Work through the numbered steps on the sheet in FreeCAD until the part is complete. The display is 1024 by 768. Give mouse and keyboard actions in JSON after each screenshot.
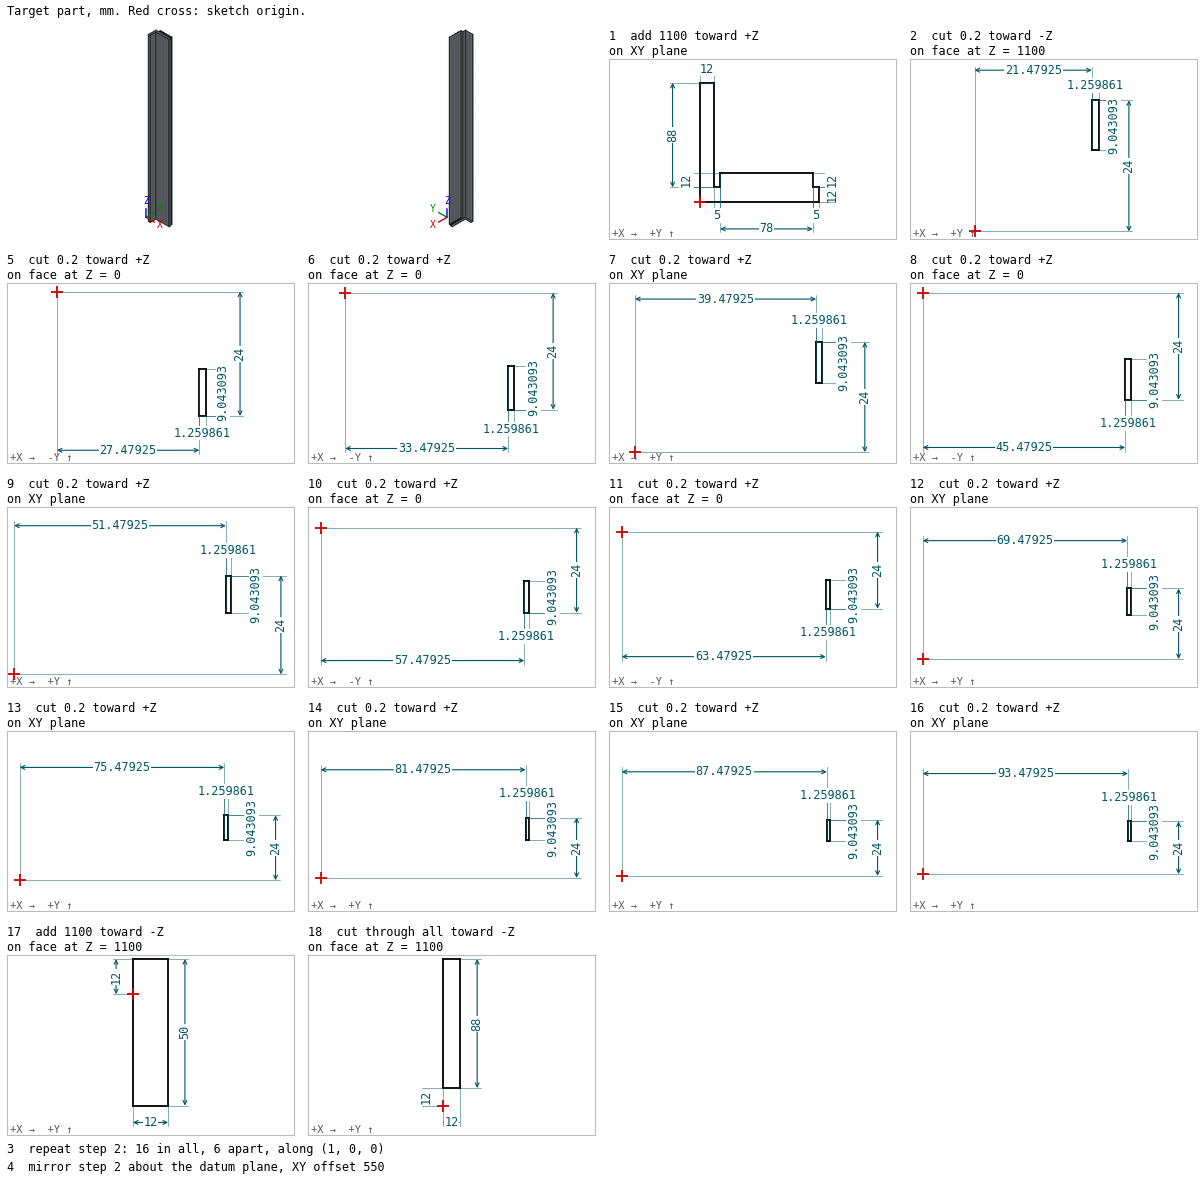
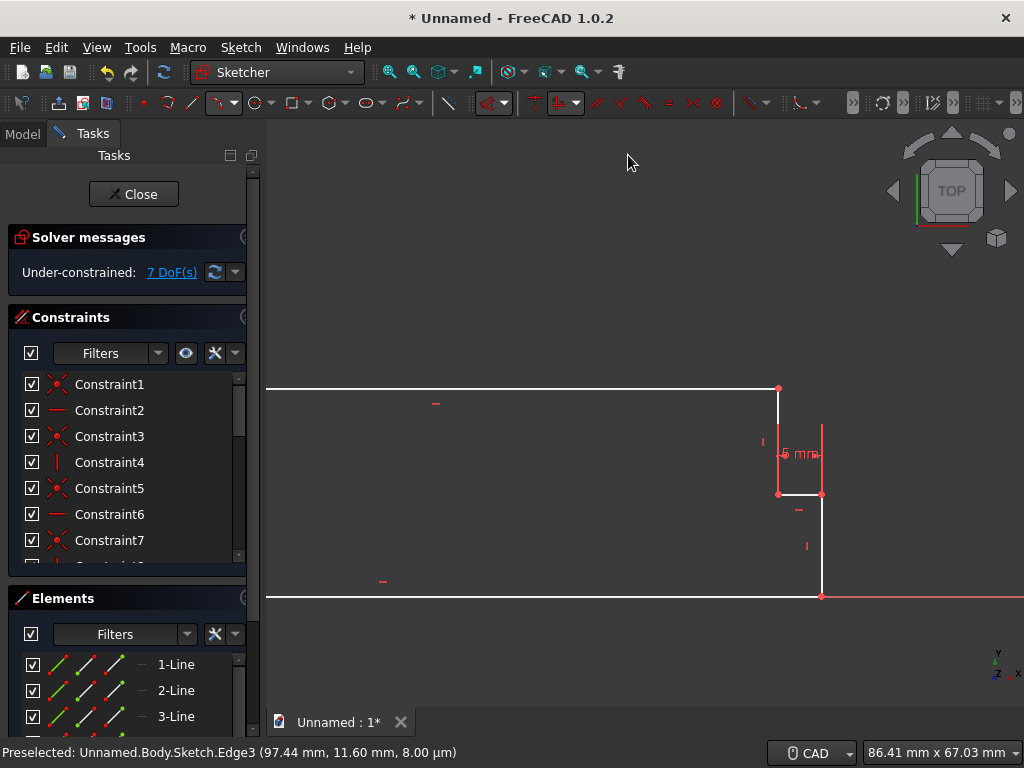
{"action": "scroll", "coordinate": [734, 621], "scroll_direction": "down", "scroll_amount": 4}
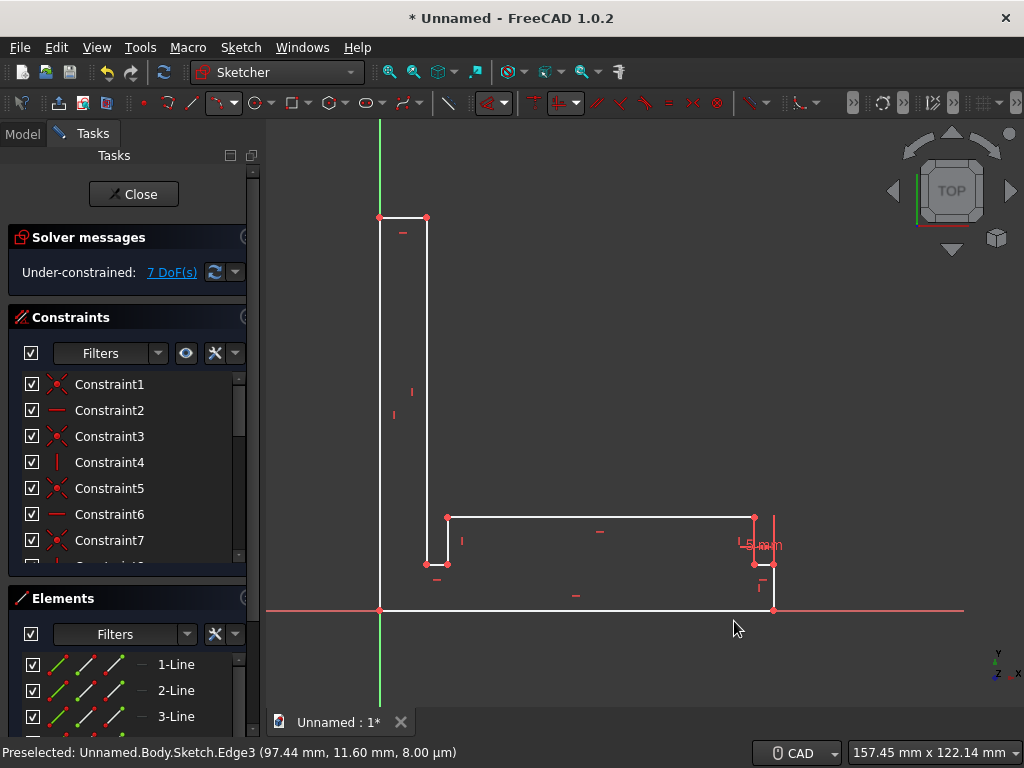
{"action": "scroll", "coordinate": [441, 565], "scroll_direction": "up", "scroll_amount": 4}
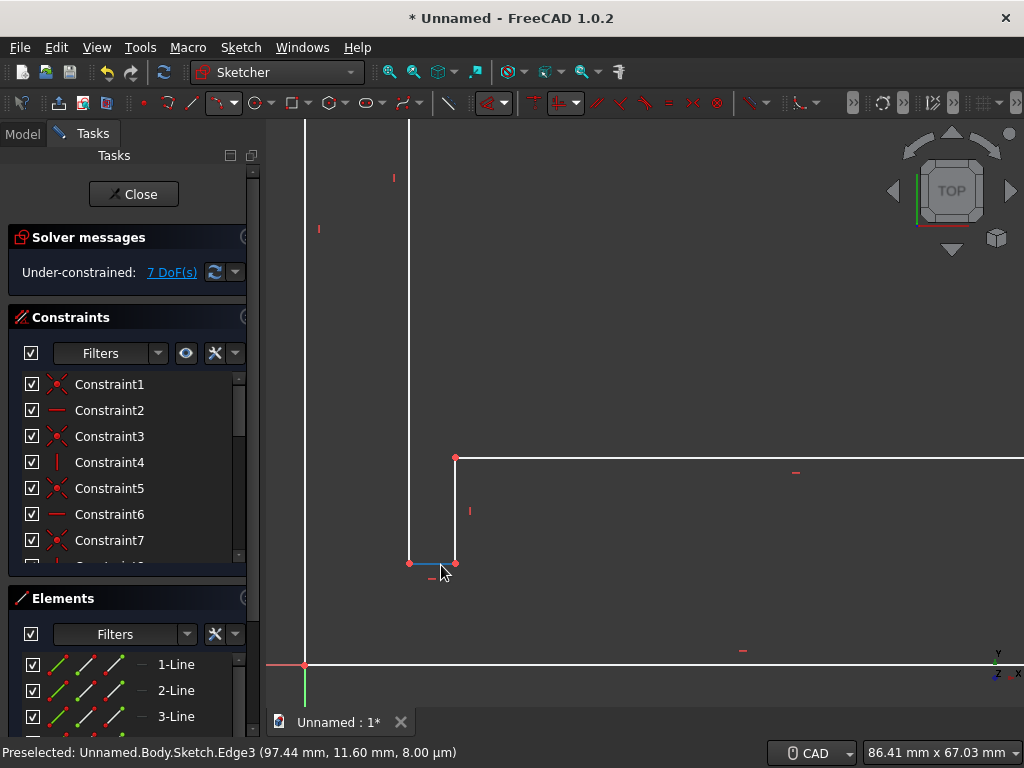
{"action": "left_click", "coordinate": [441, 564]}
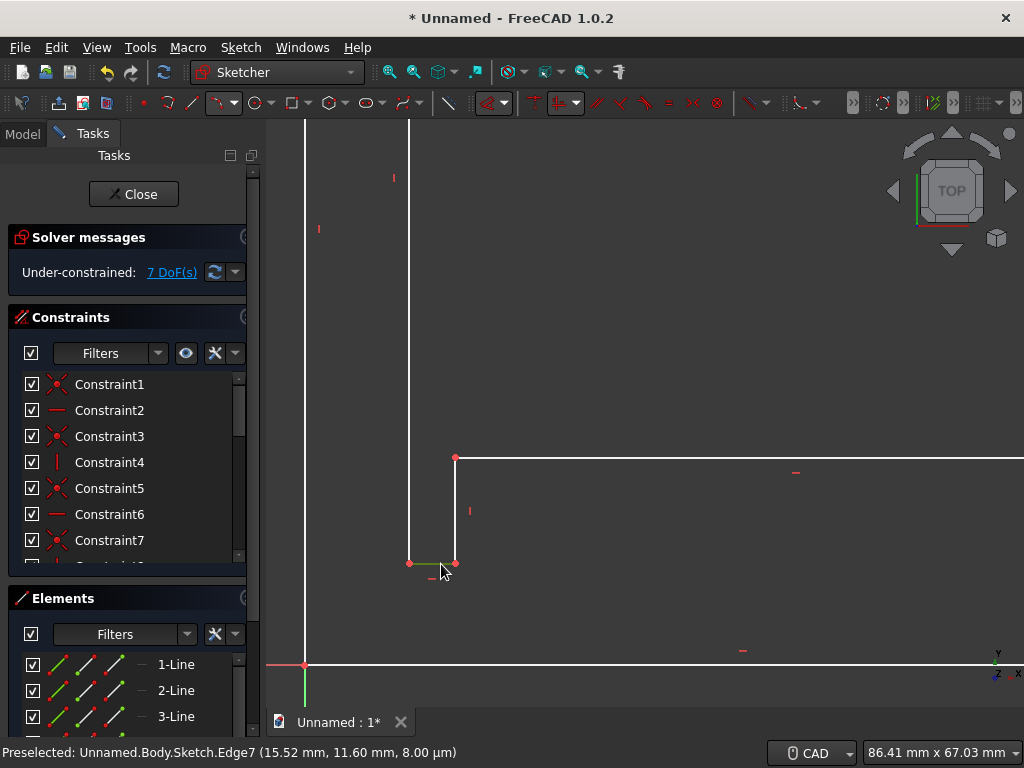
{"action": "key", "text": "l"}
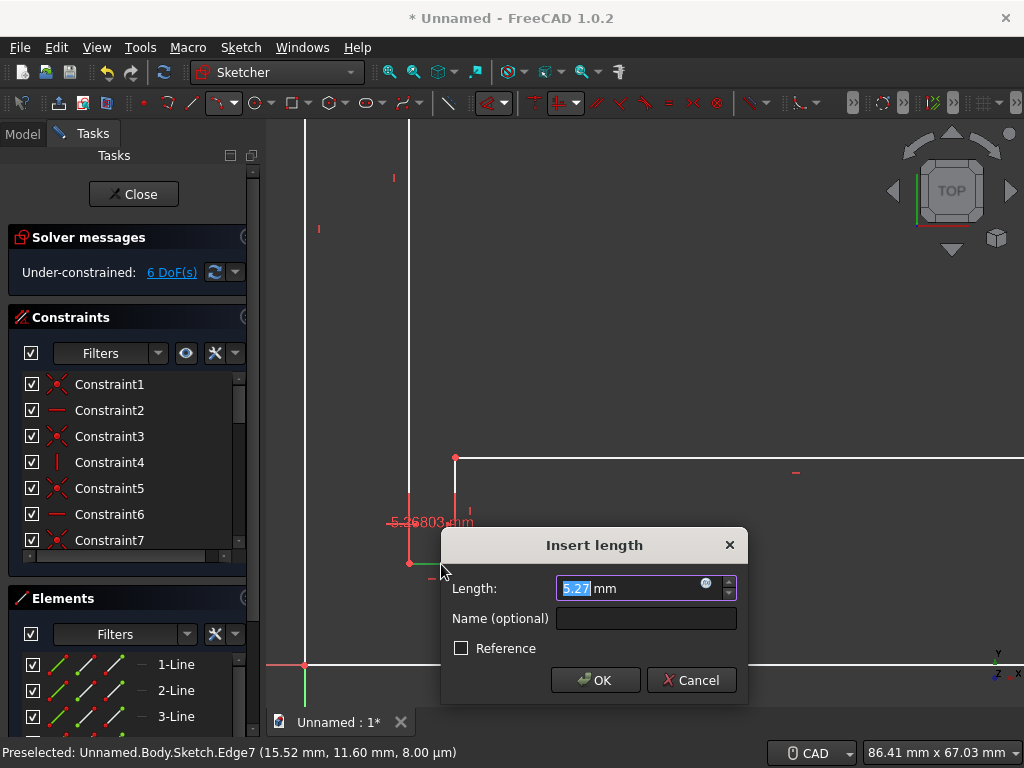
{"action": "type", "text": "5"}
{"action": "key", "text": "Return"}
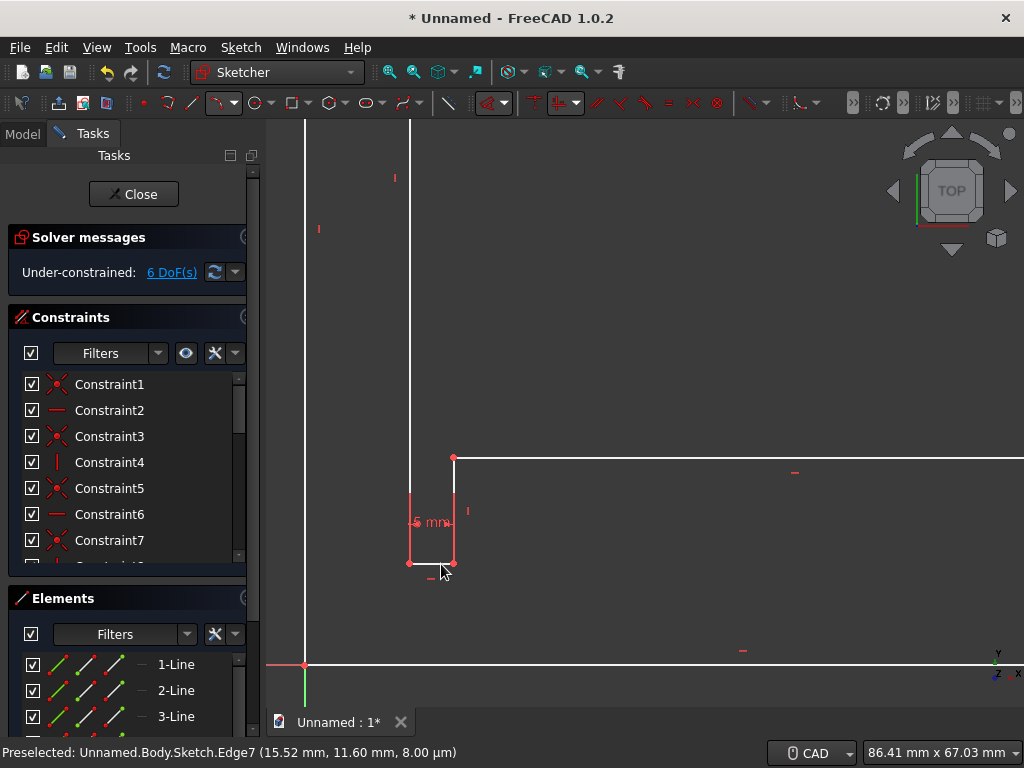
{"action": "scroll", "coordinate": [440, 565], "scroll_direction": "down", "scroll_amount": 4}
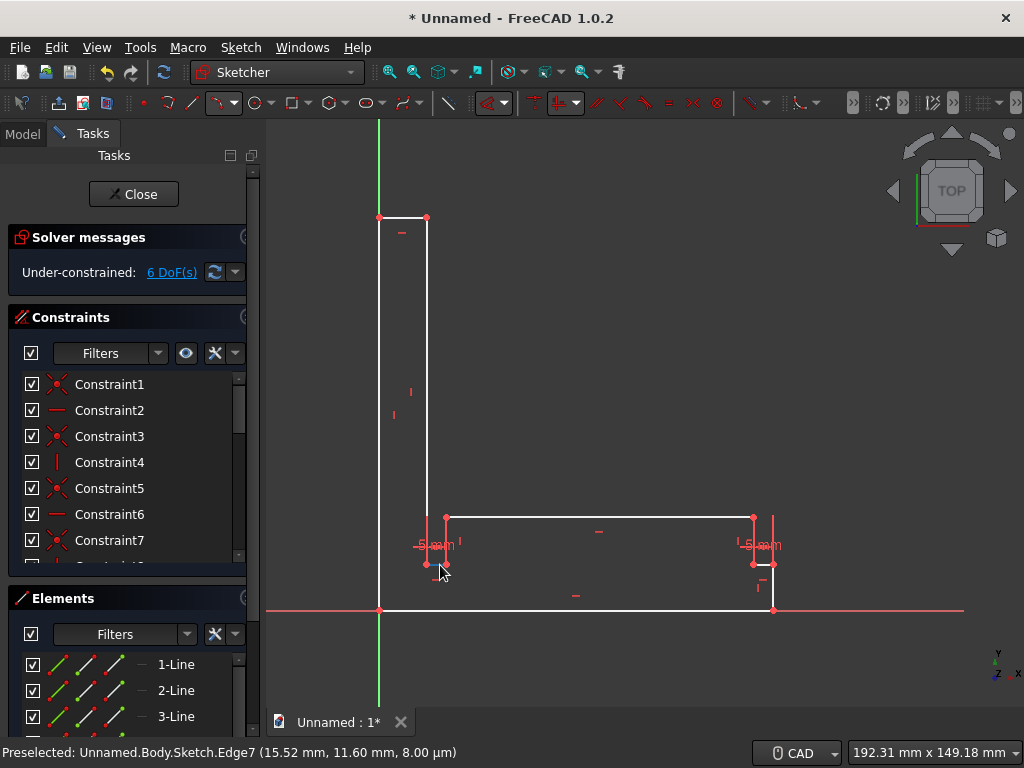
{"action": "left_click", "coordinate": [773, 597]}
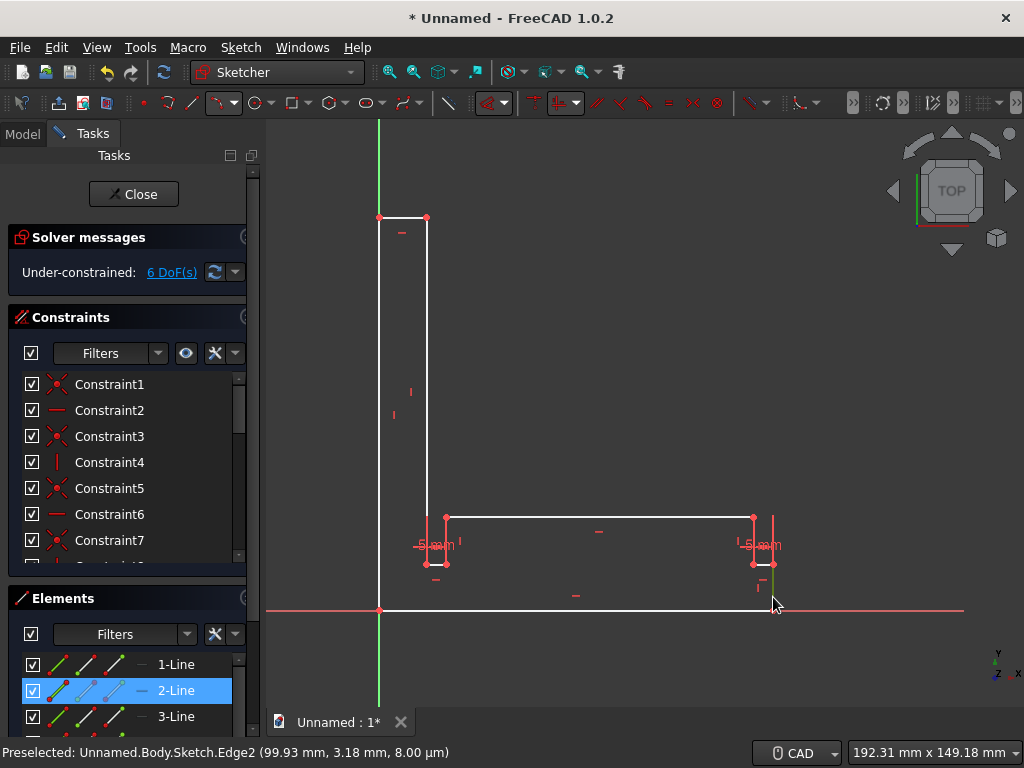
{"action": "left_click", "coordinate": [506, 104]}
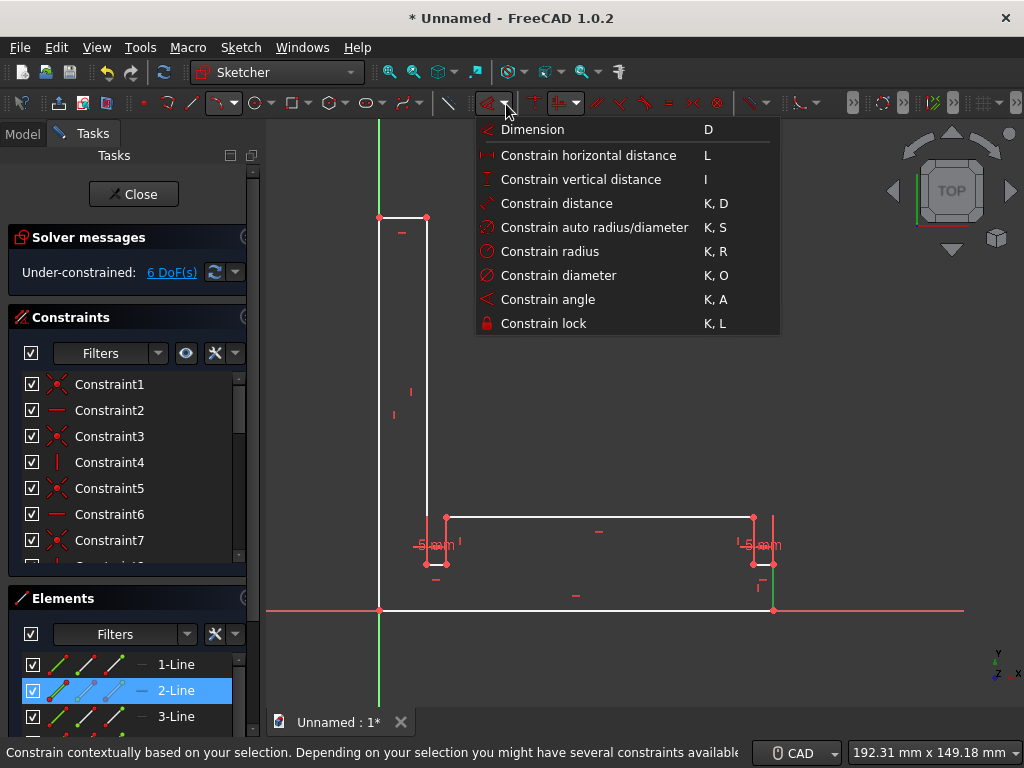
{"action": "left_click", "coordinate": [628, 179]}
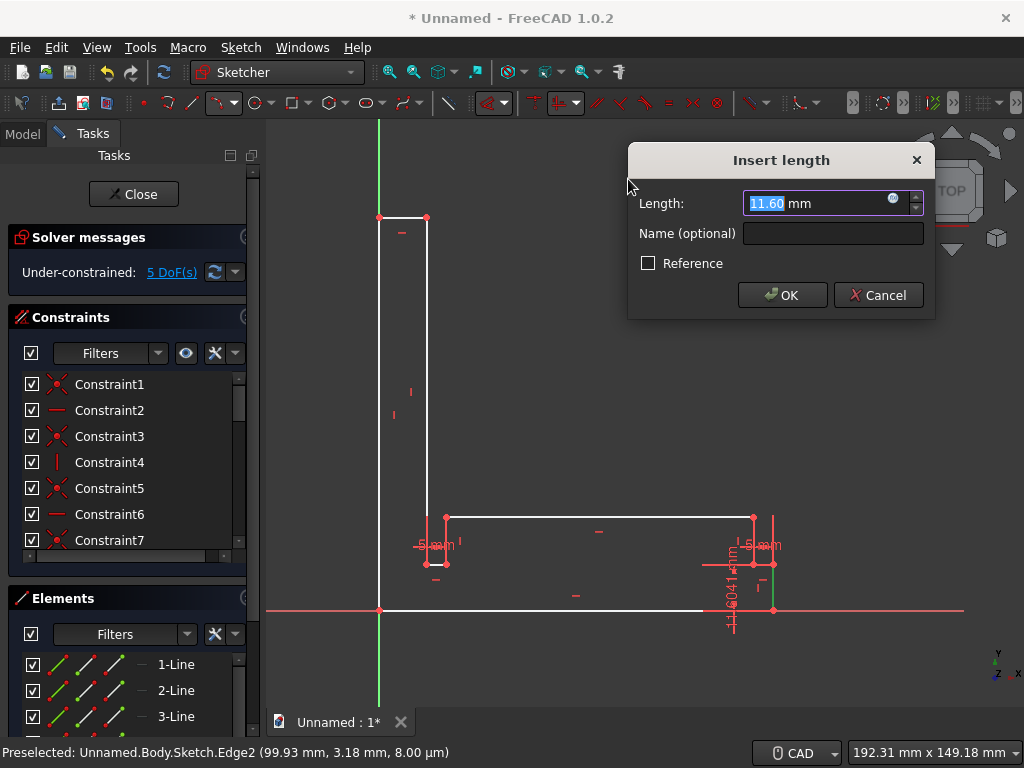
{"action": "type", "text": "12"}
{"action": "key", "text": "Return"}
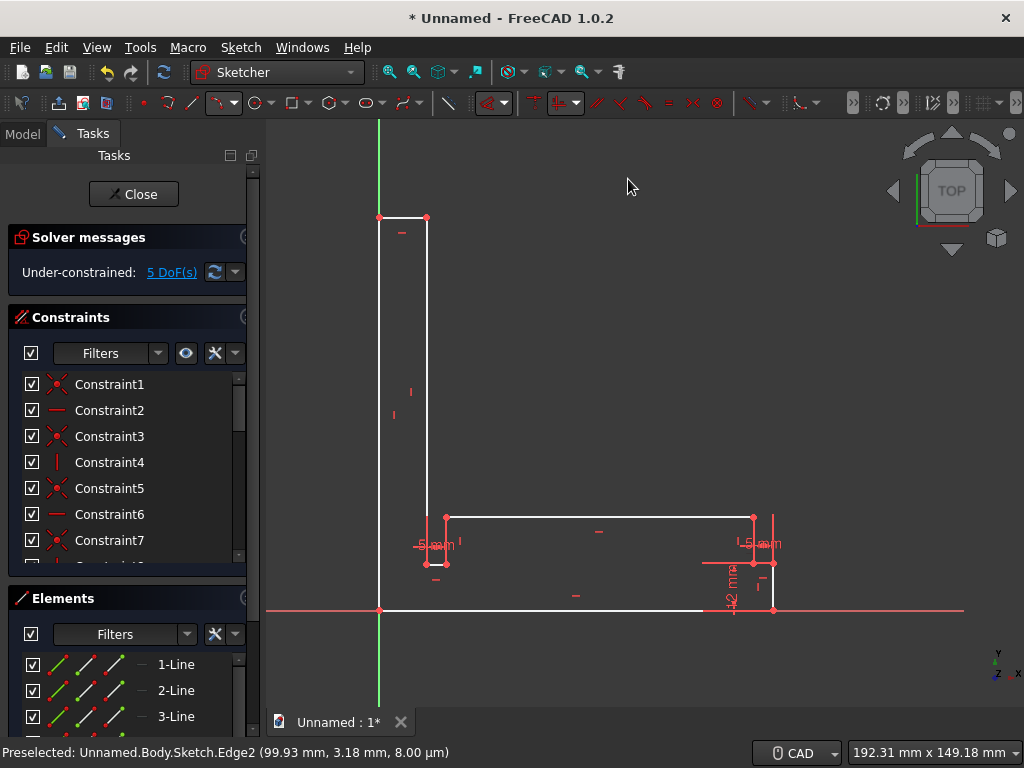
{"action": "left_click", "coordinate": [754, 531]}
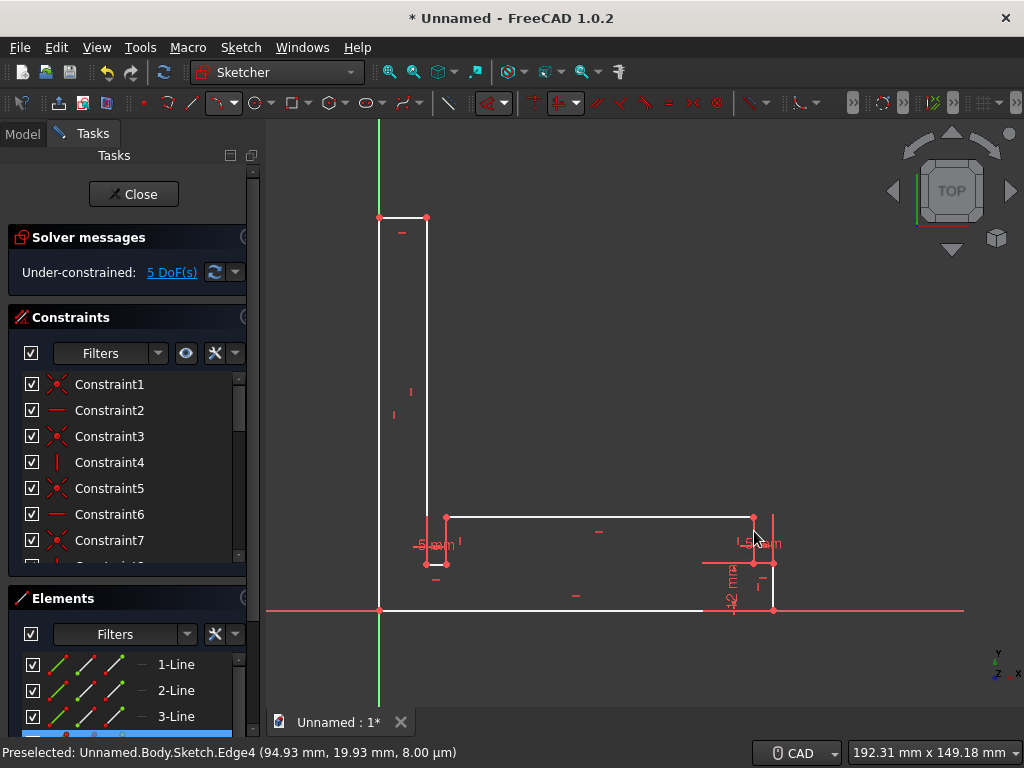
{"action": "left_click", "coordinate": [506, 104]}